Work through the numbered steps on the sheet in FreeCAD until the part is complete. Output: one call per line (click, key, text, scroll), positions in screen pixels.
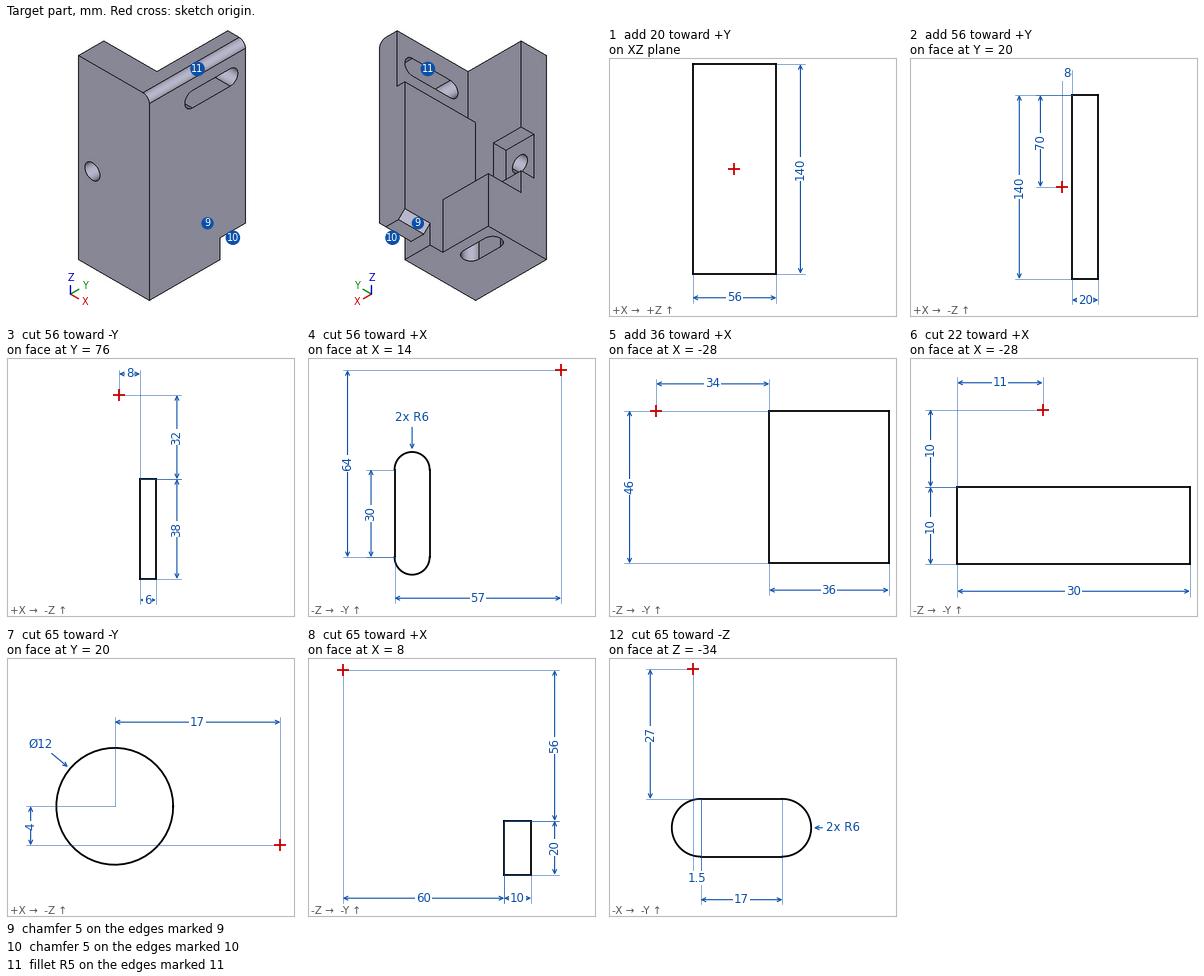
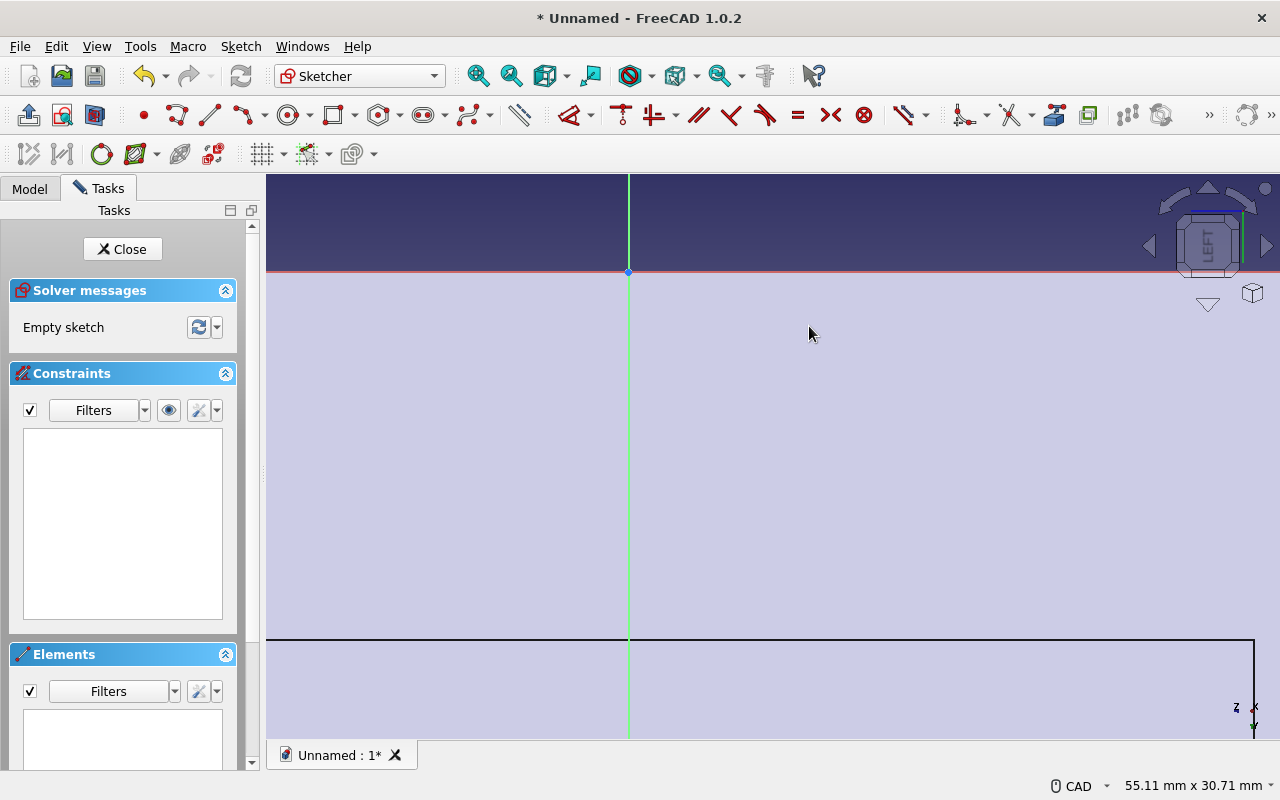
click(332, 116)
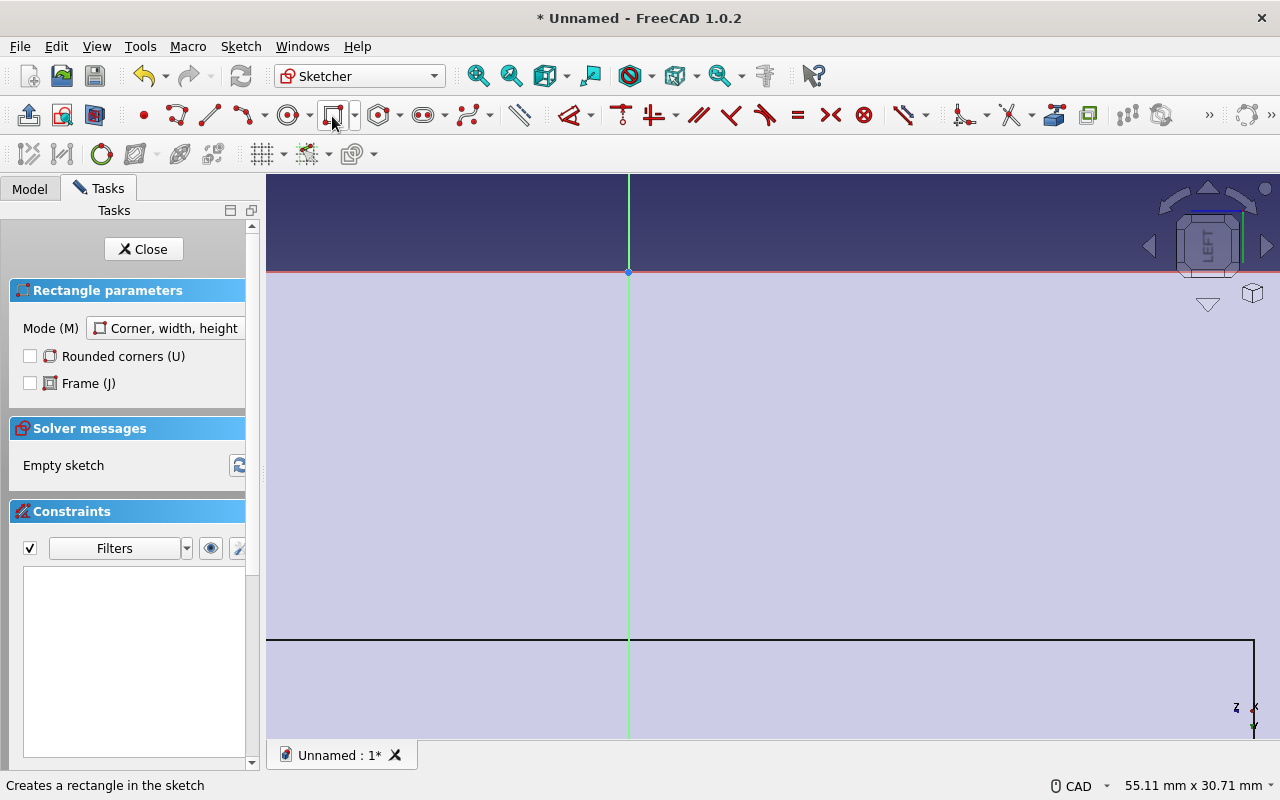
click(426, 456)
click(978, 640)
key(Escape)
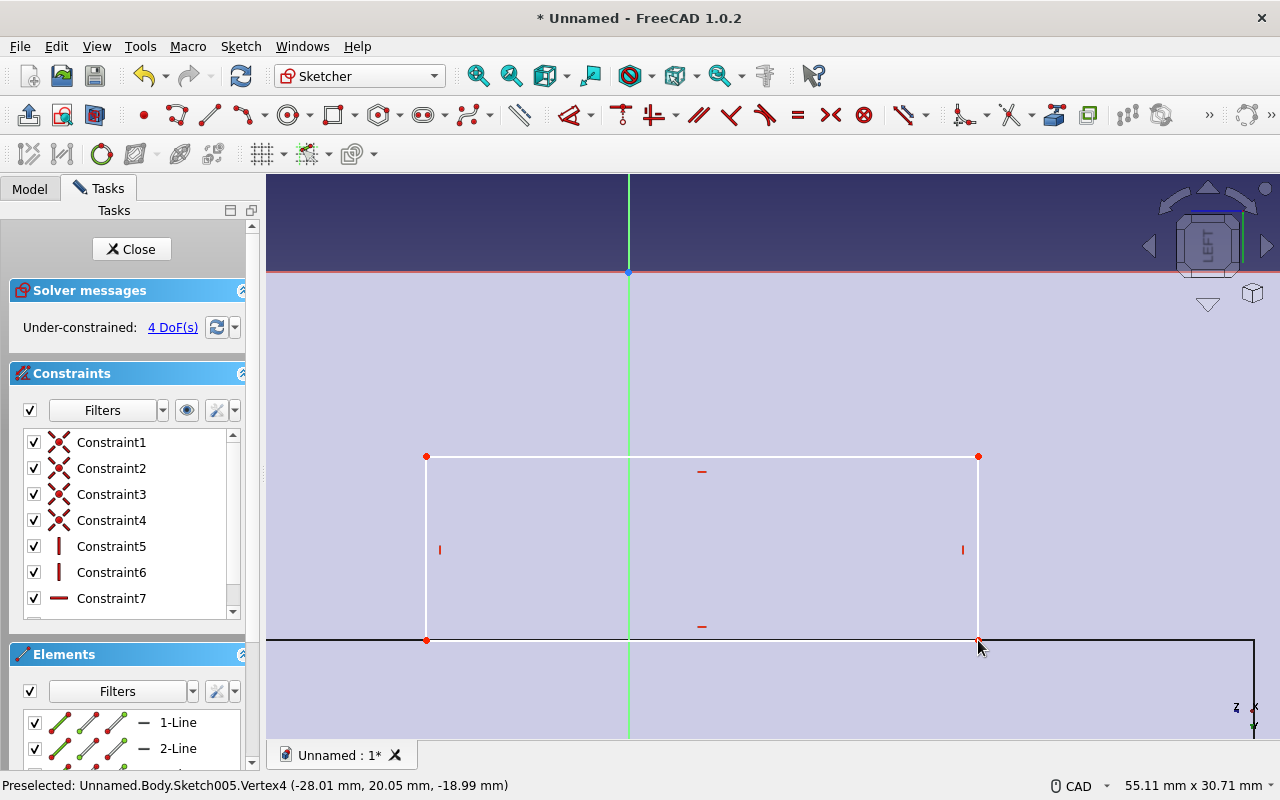
click(568, 116)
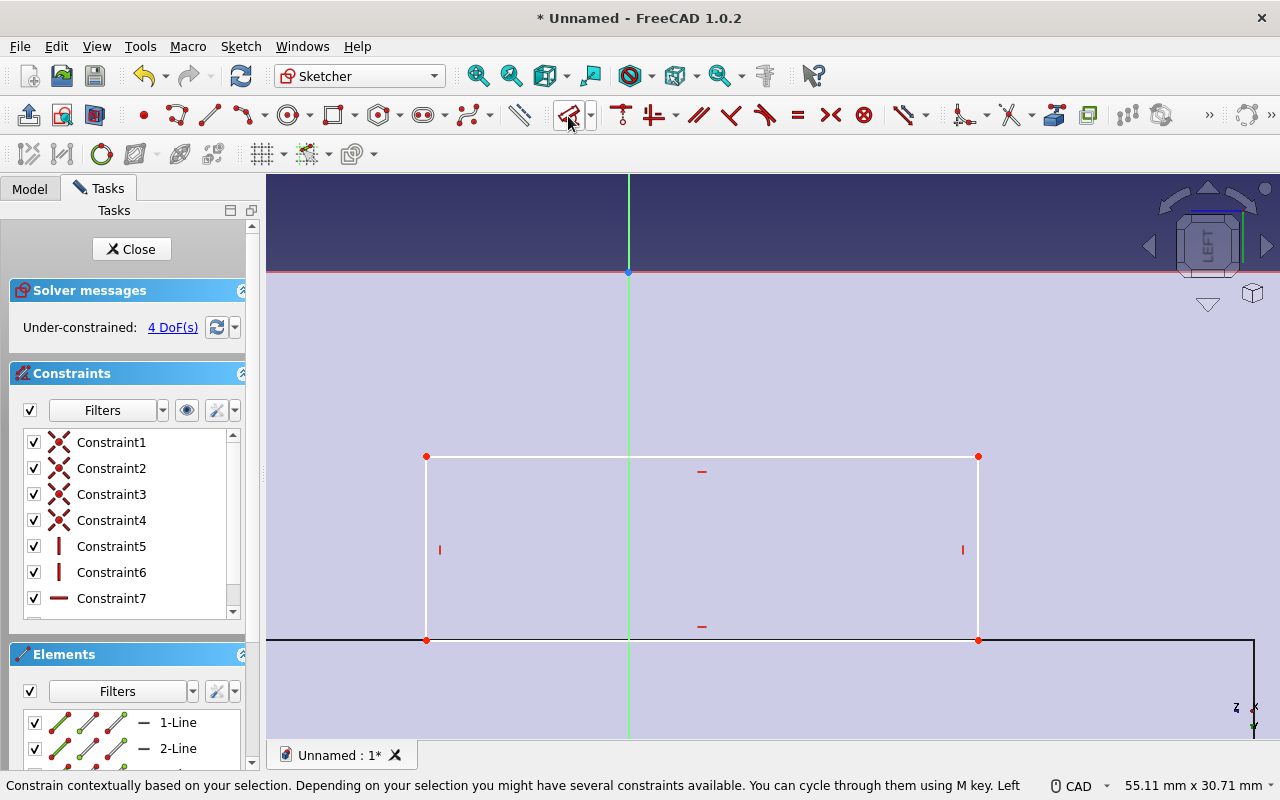
click(426, 512)
click(392, 549)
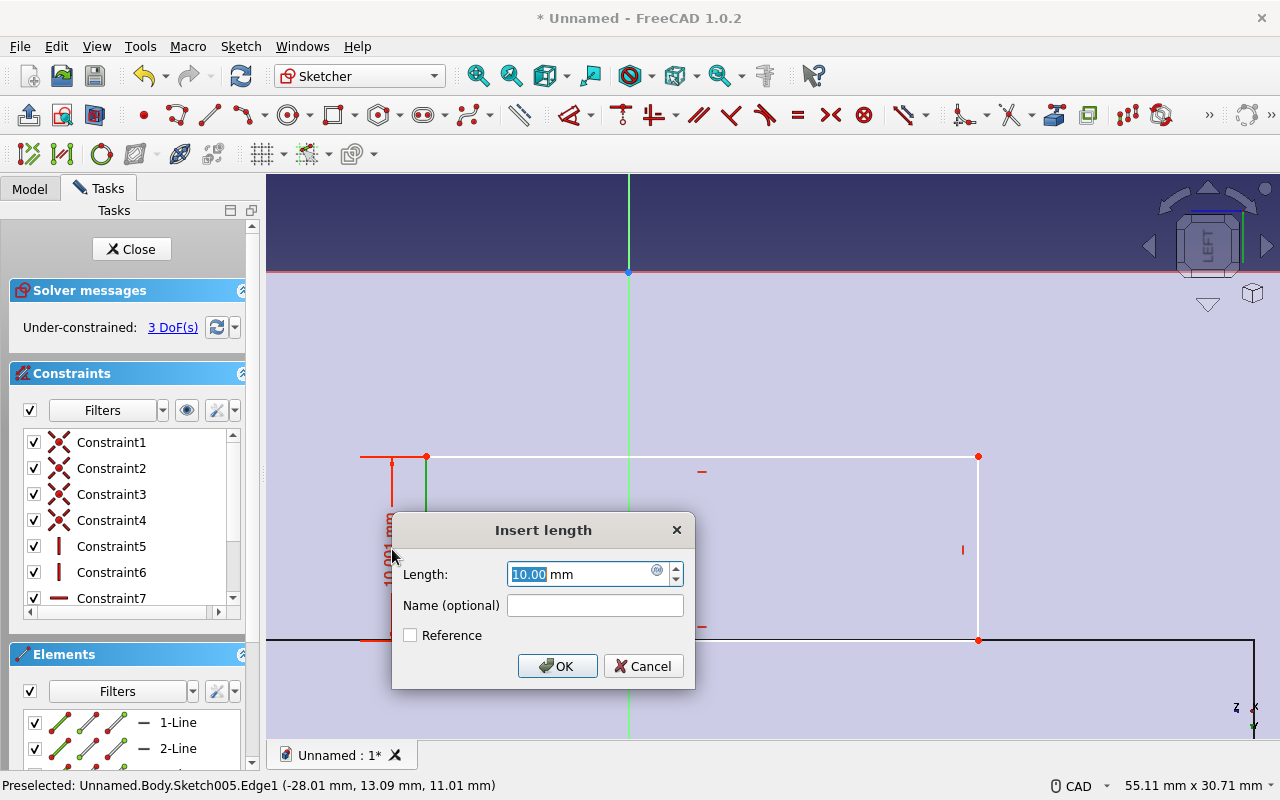
text(10)
key(Return)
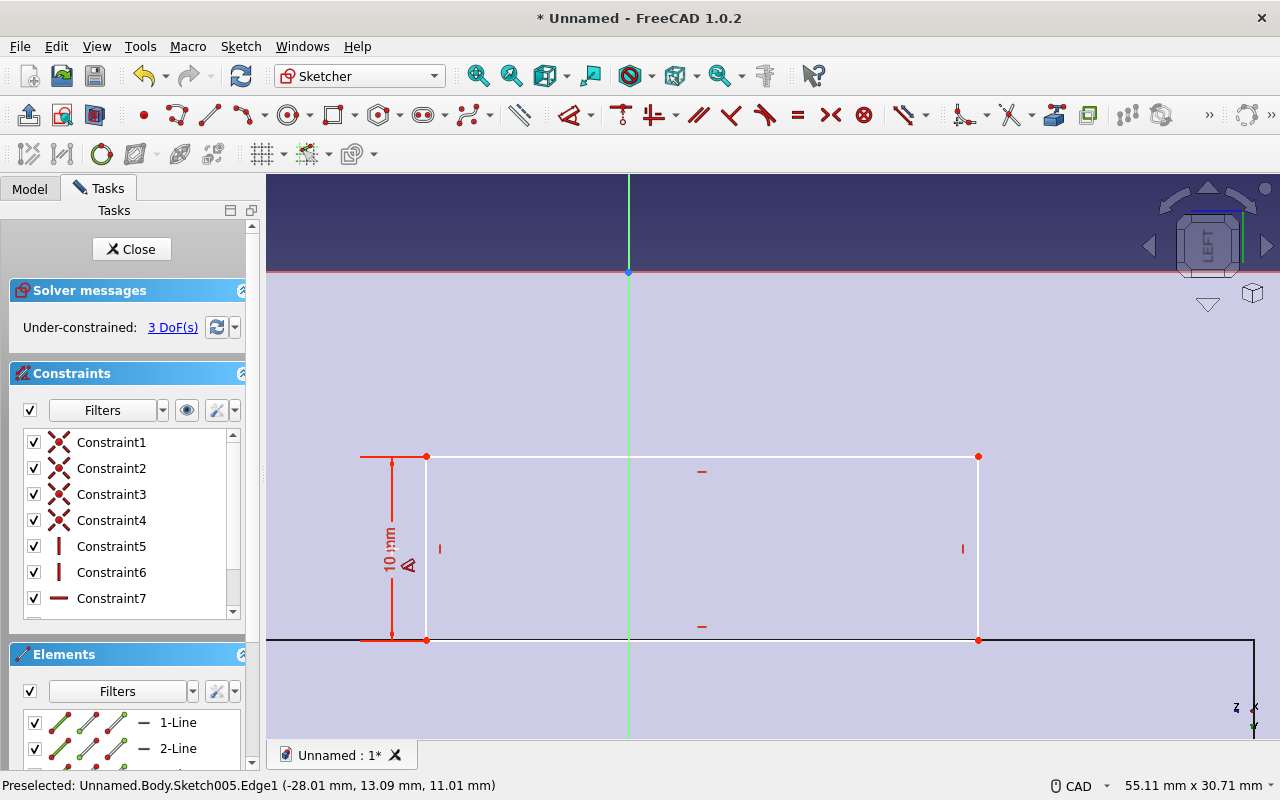
click(592, 641)
click(702, 675)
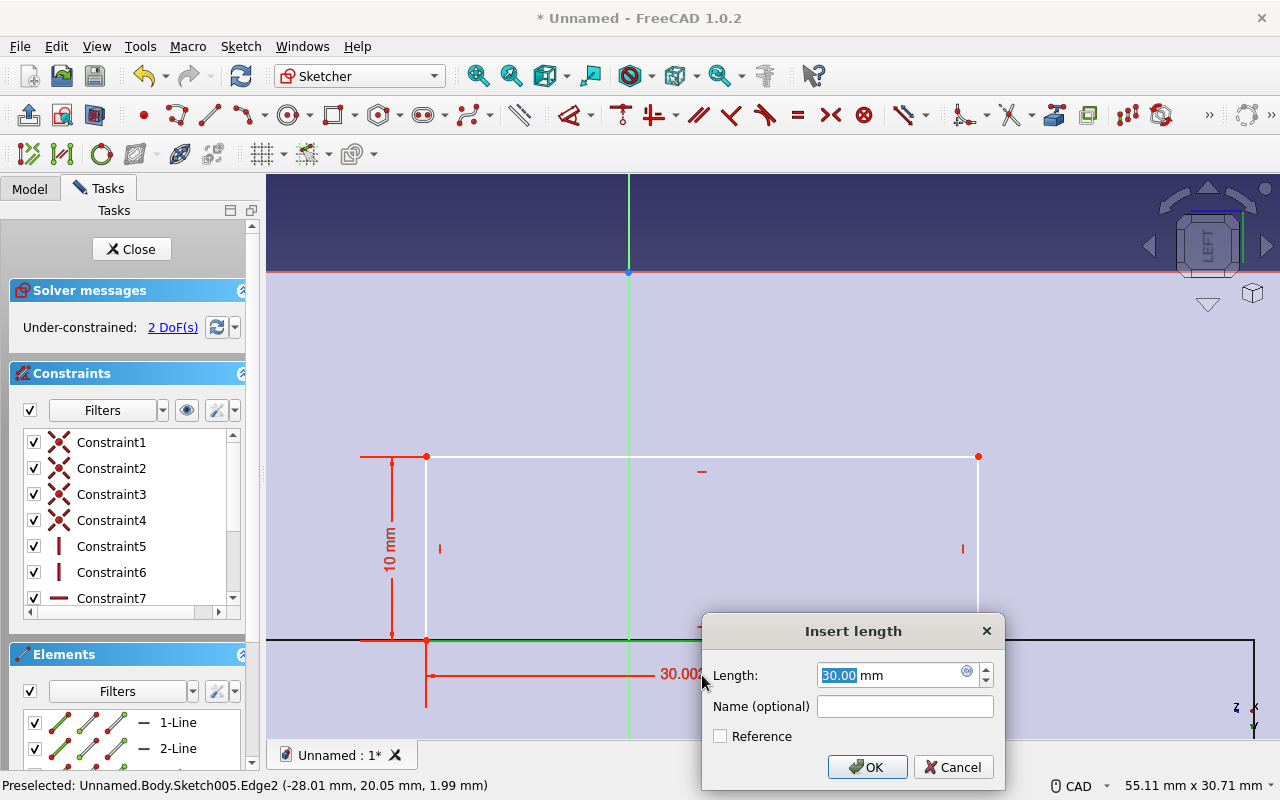
text(30)
key(Return)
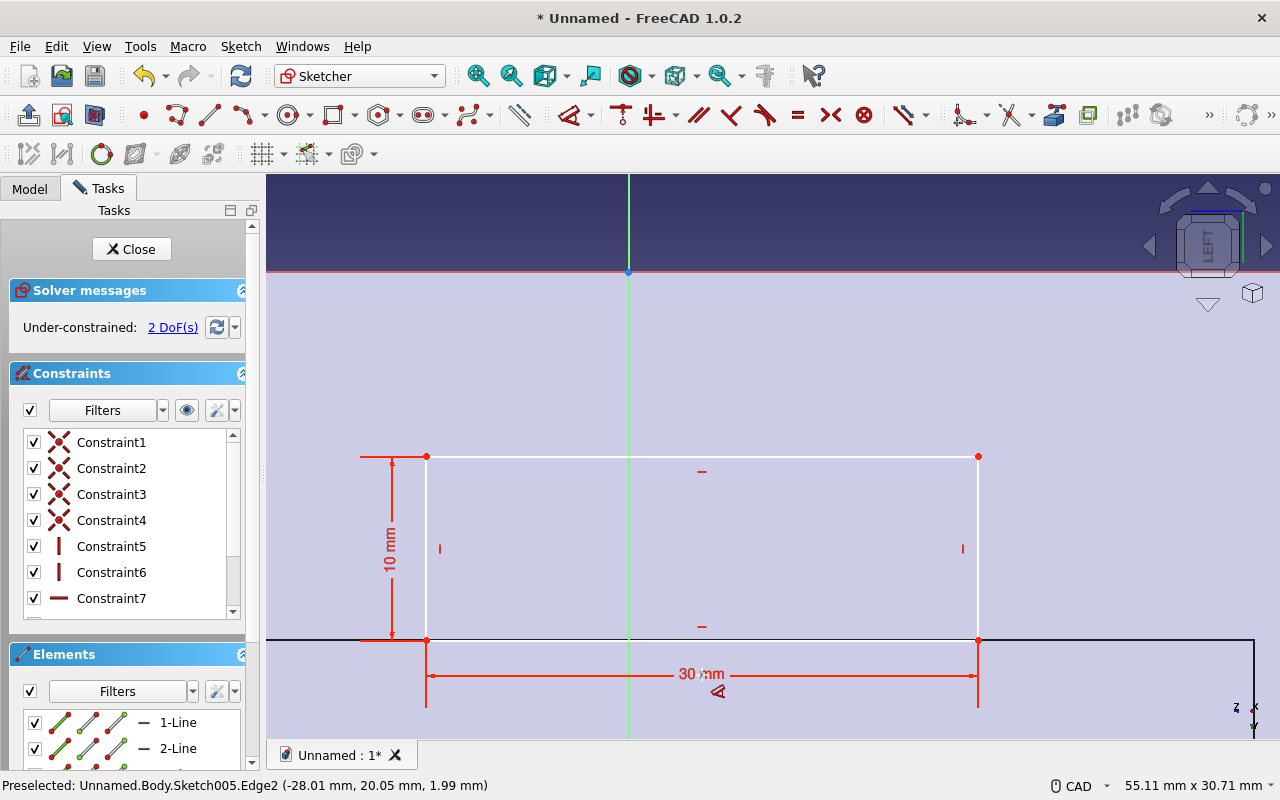
click(426, 457)
click(527, 238)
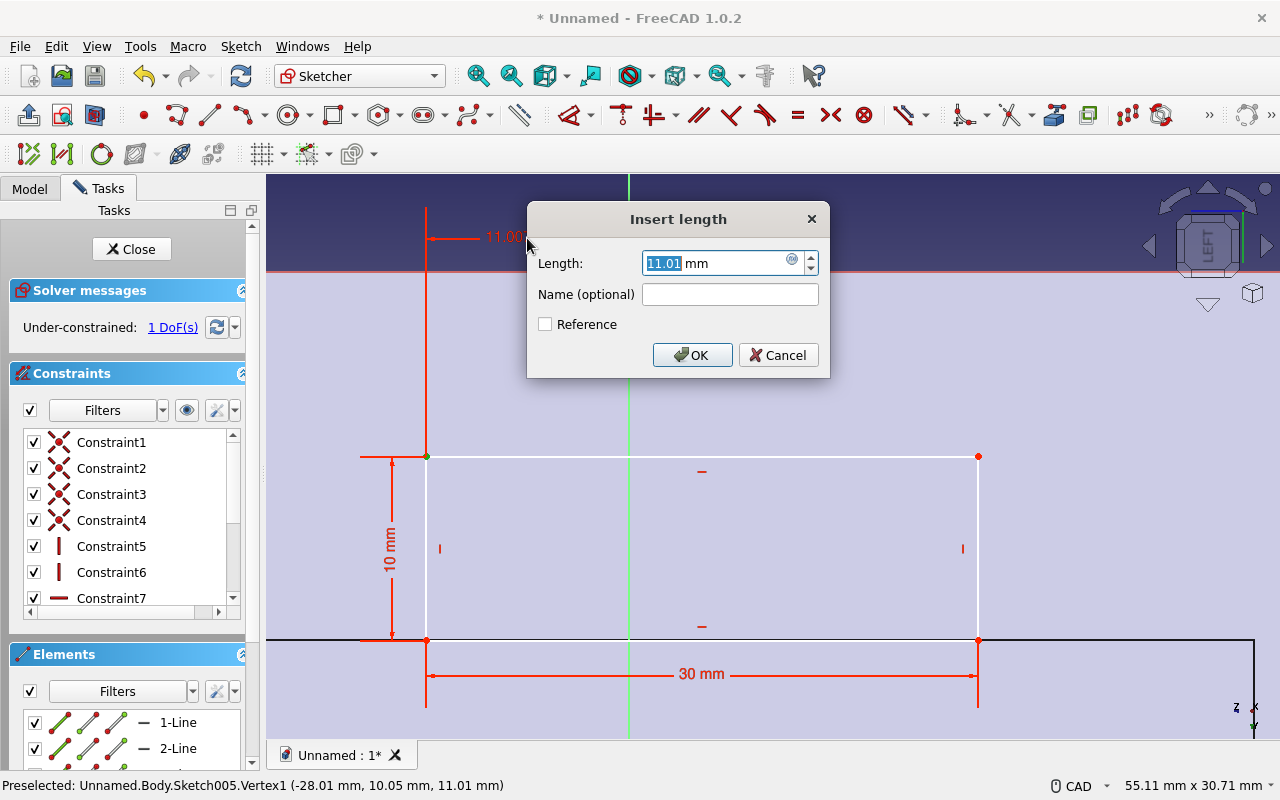
text(11)
key(Return)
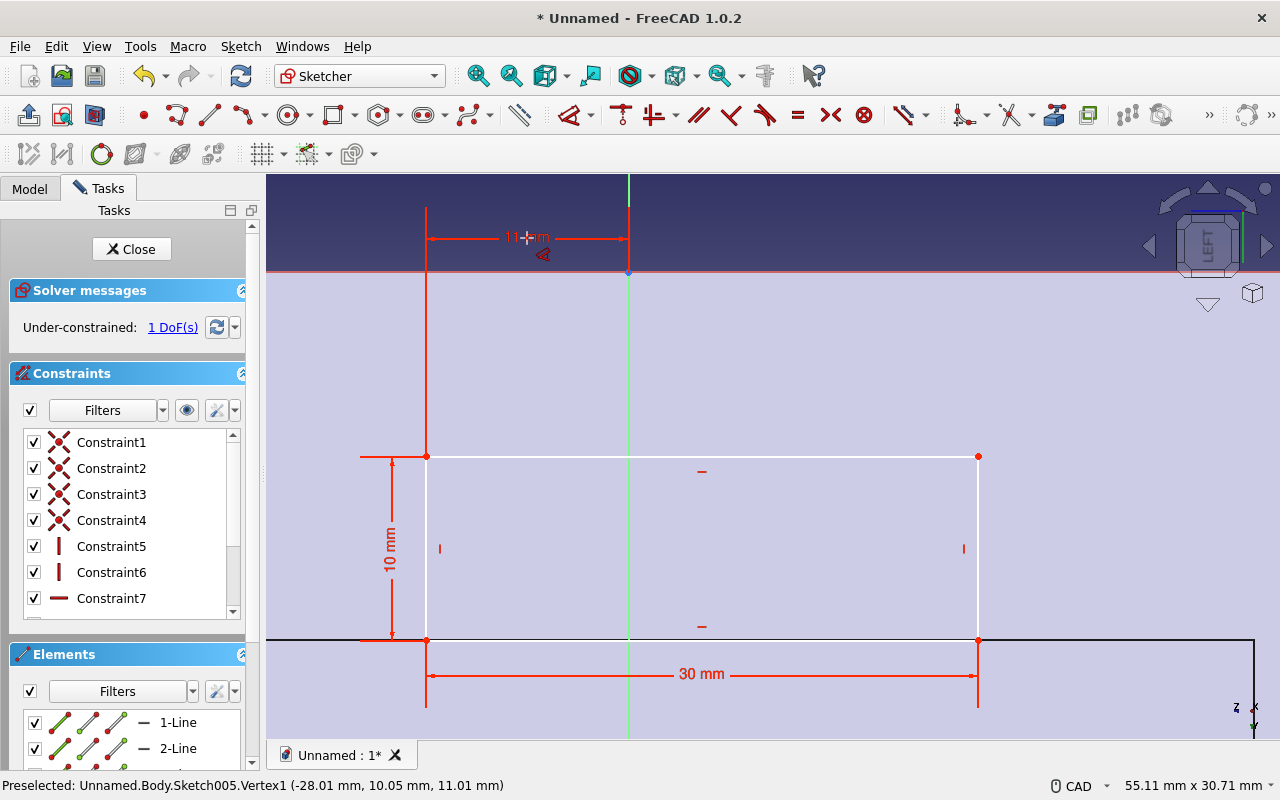
click(426, 457)
click(392, 365)